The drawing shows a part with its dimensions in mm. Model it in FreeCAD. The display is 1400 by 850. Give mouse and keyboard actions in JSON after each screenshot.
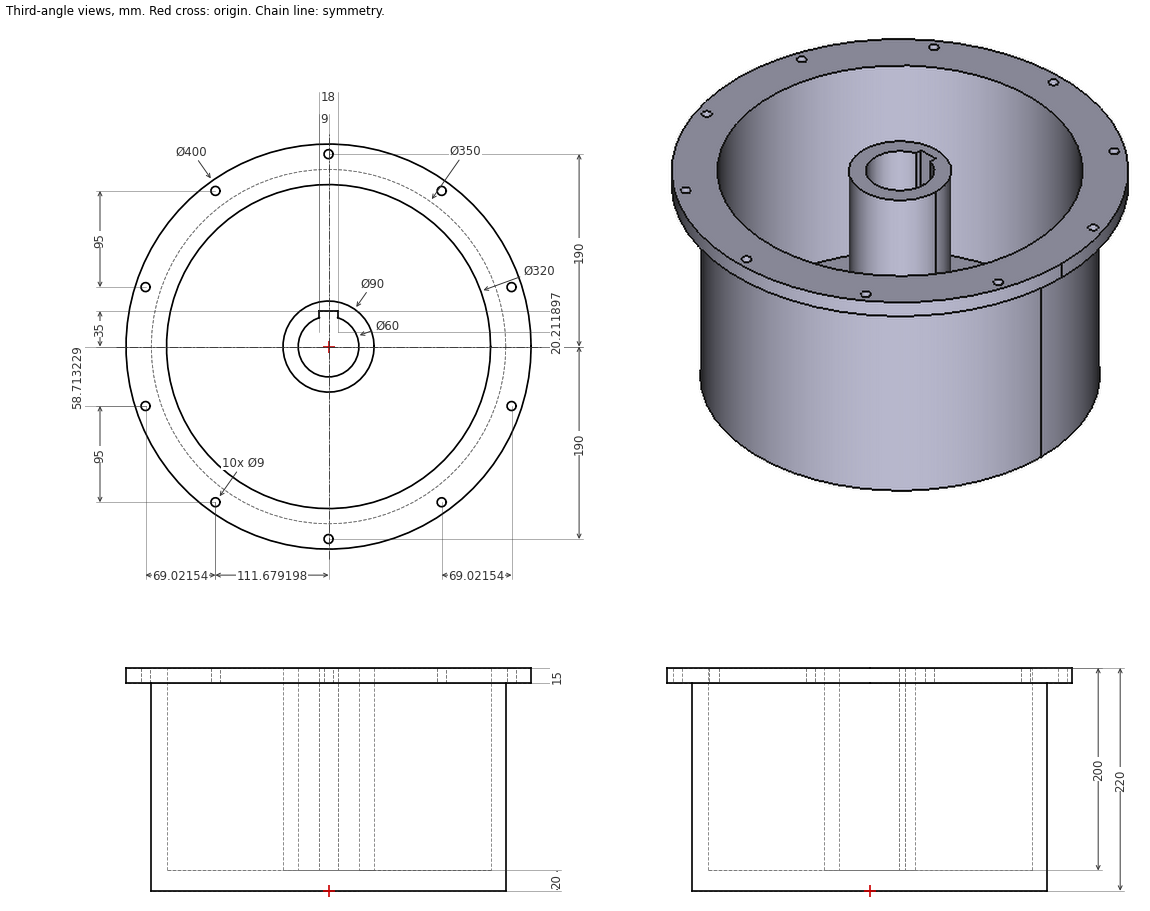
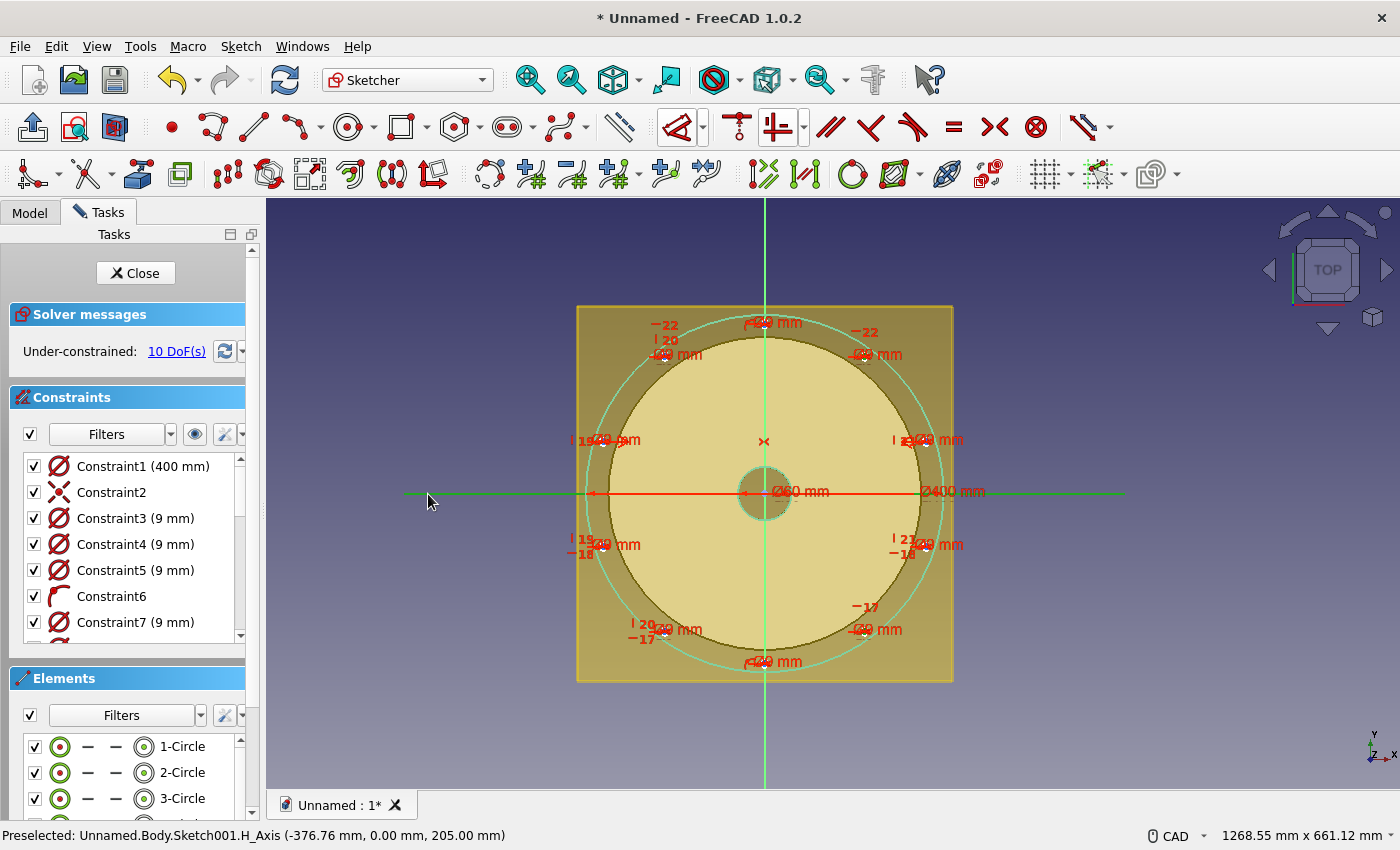
{"action": "left_click", "coordinate": [995, 128]}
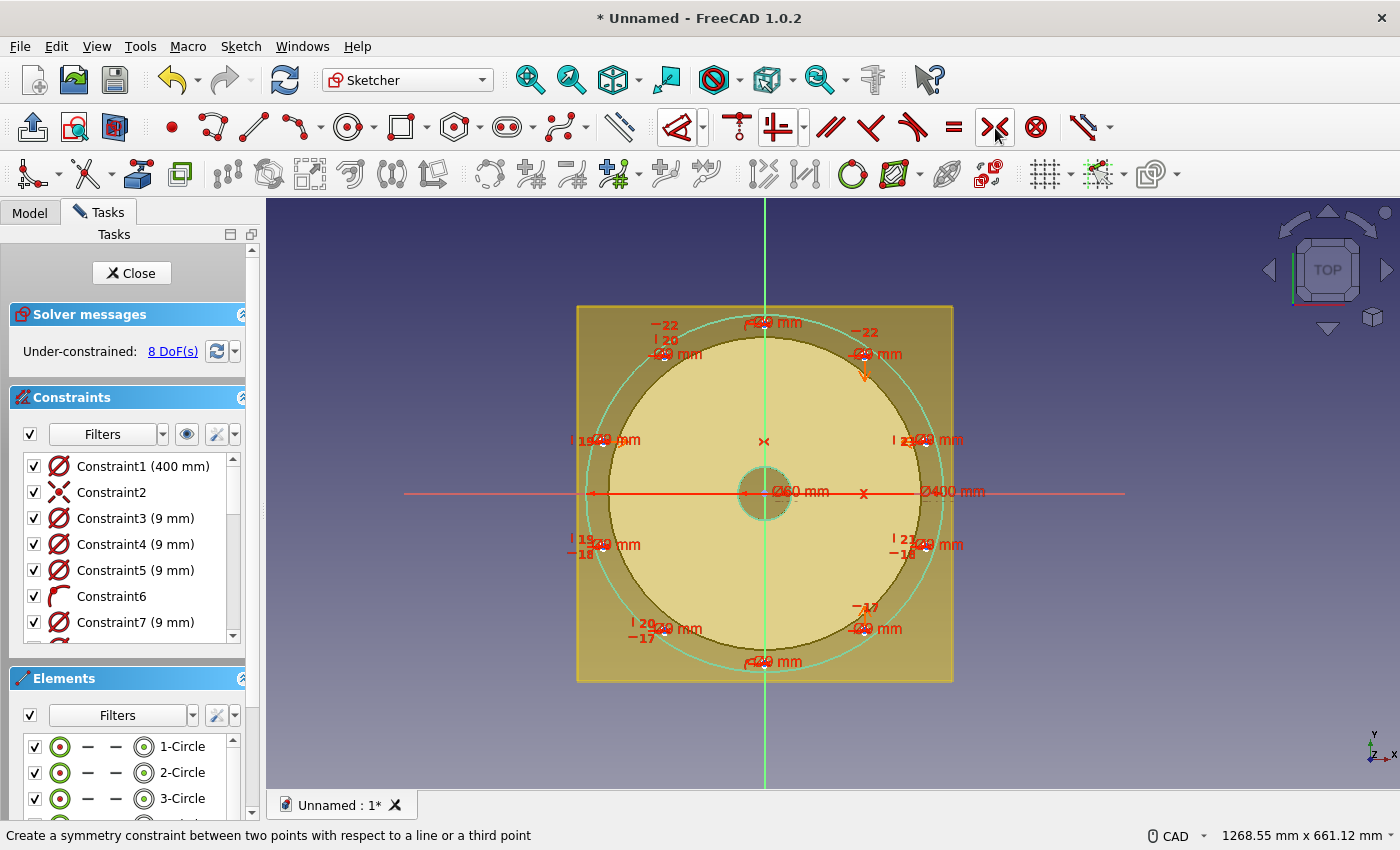
{"action": "left_click", "coordinate": [676, 128]}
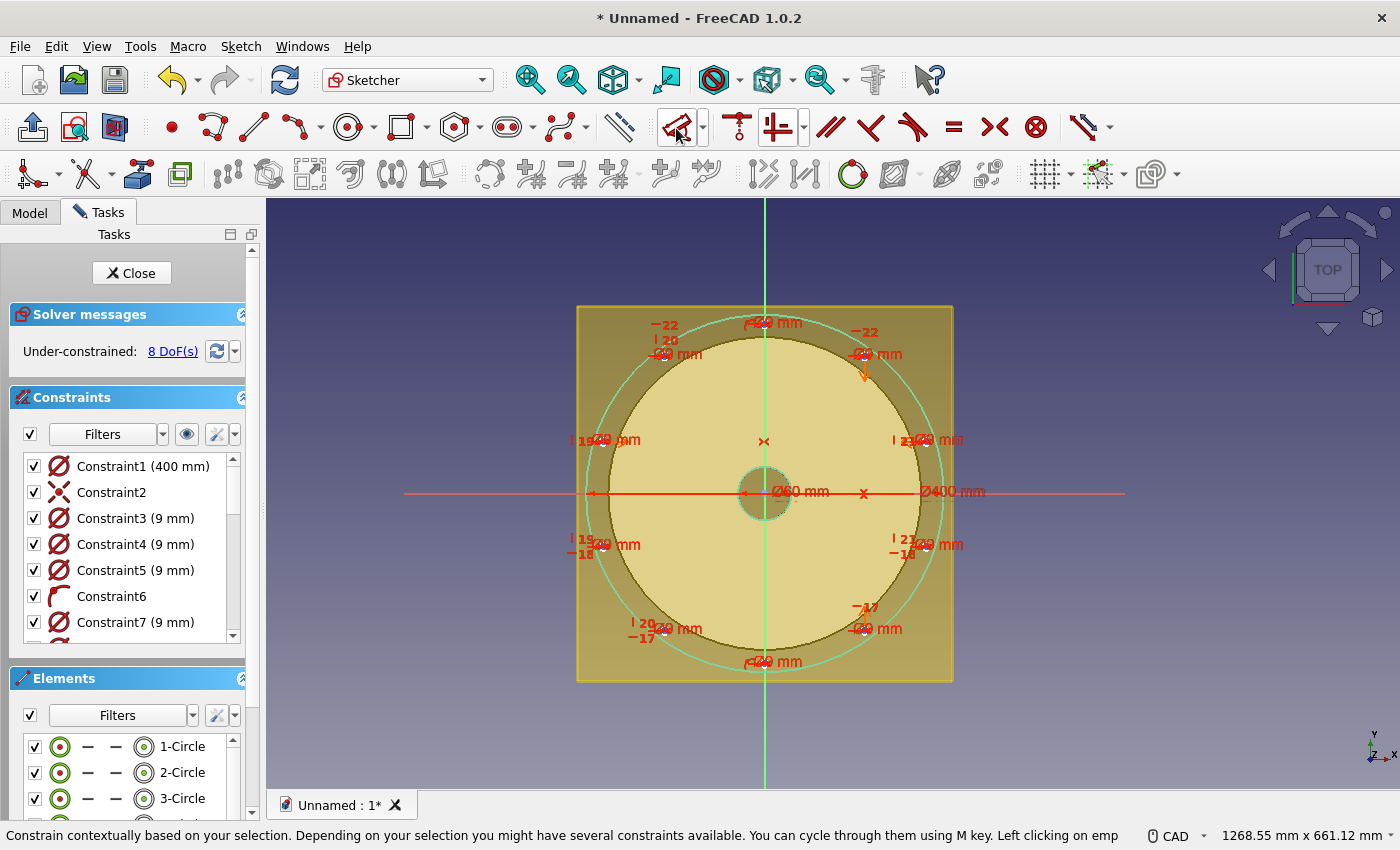
{"action": "left_click", "coordinate": [765, 664]}
{"action": "left_click", "coordinate": [799, 579]}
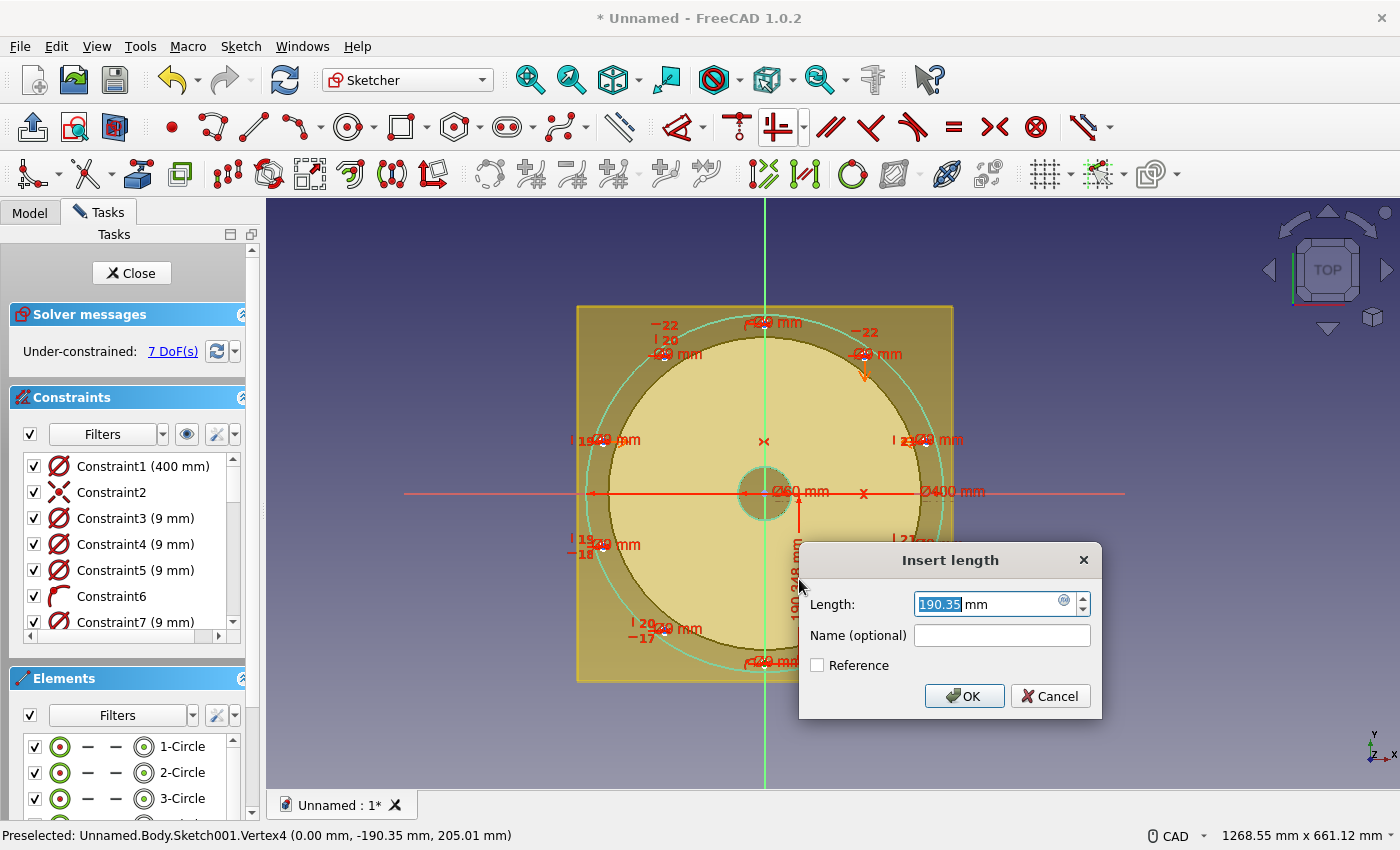
{"action": "type", "text": "190"}
{"action": "key", "text": "Return"}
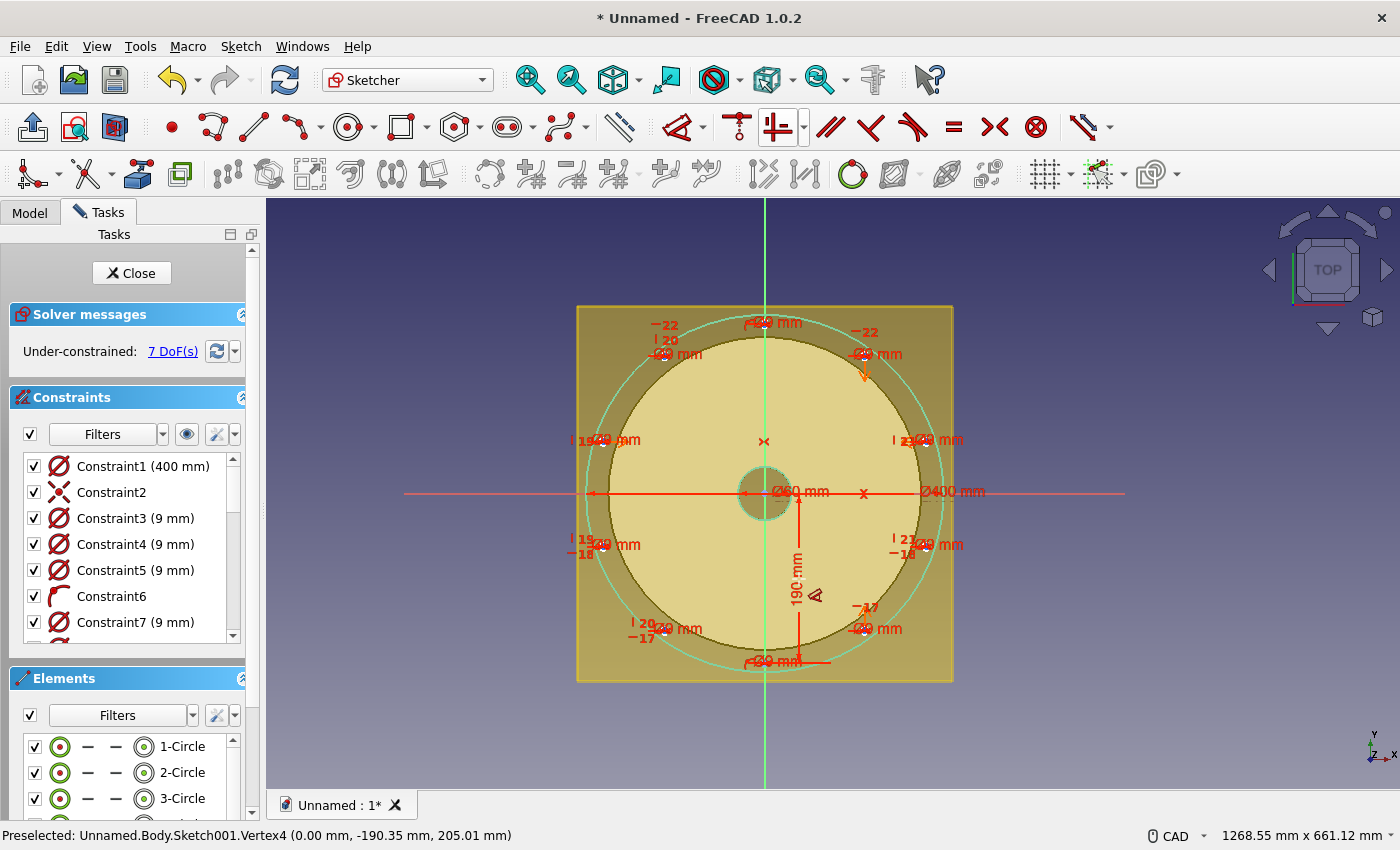
{"action": "left_click", "coordinate": [765, 324]}
{"action": "left_click", "coordinate": [799, 409]}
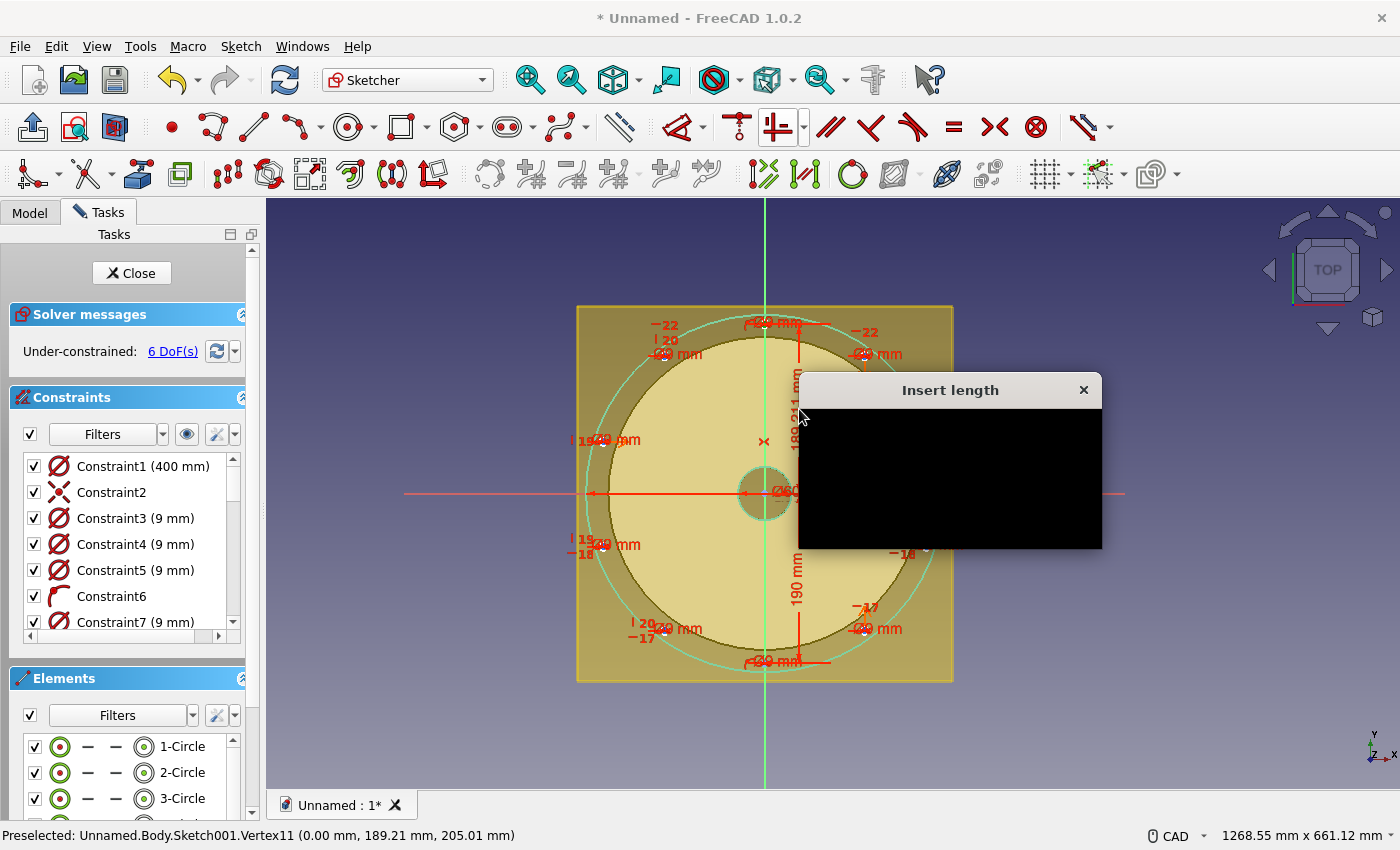
{"action": "type", "text": "190"}
{"action": "key", "text": "Return"}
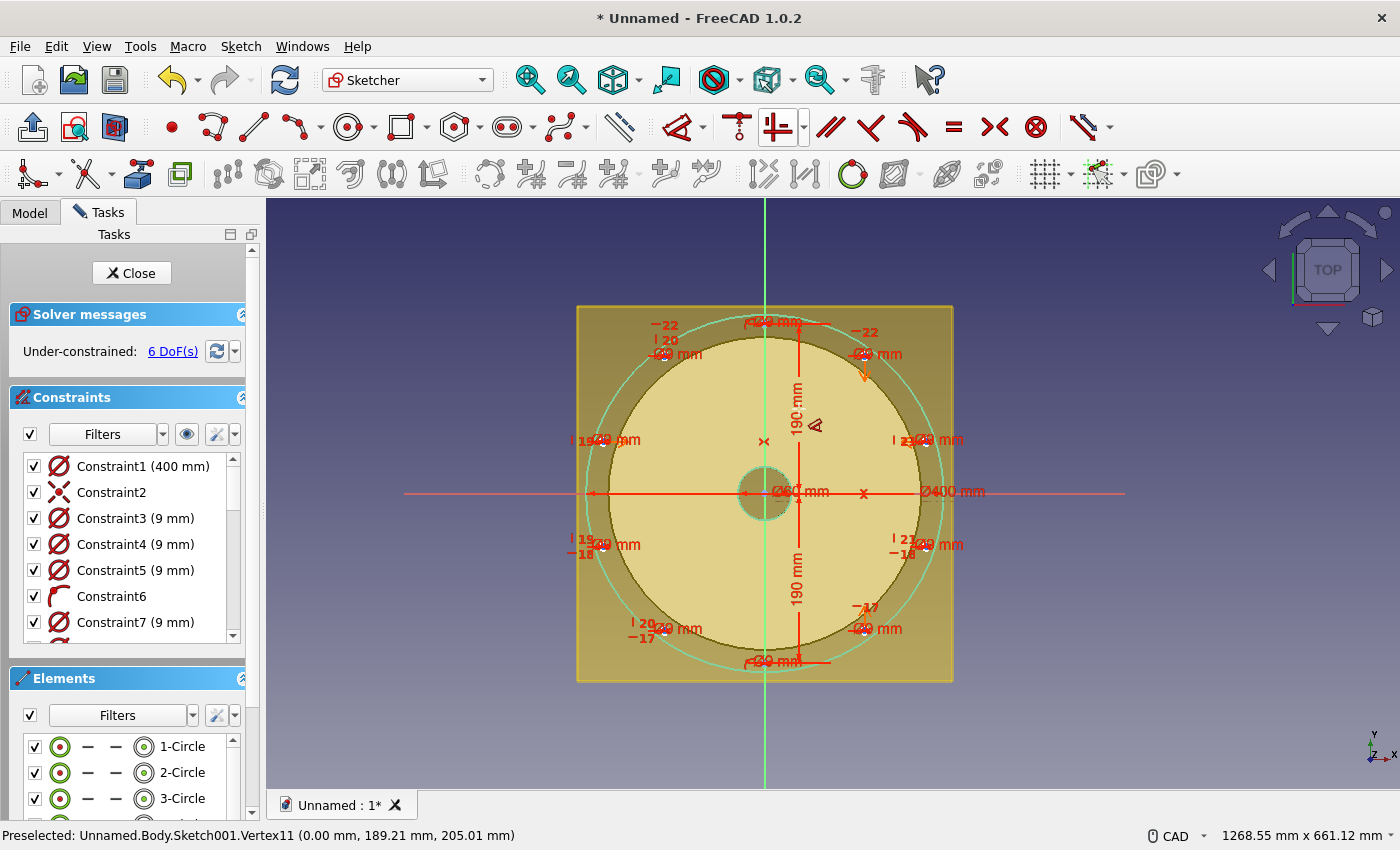
{"action": "left_click", "coordinate": [665, 631]}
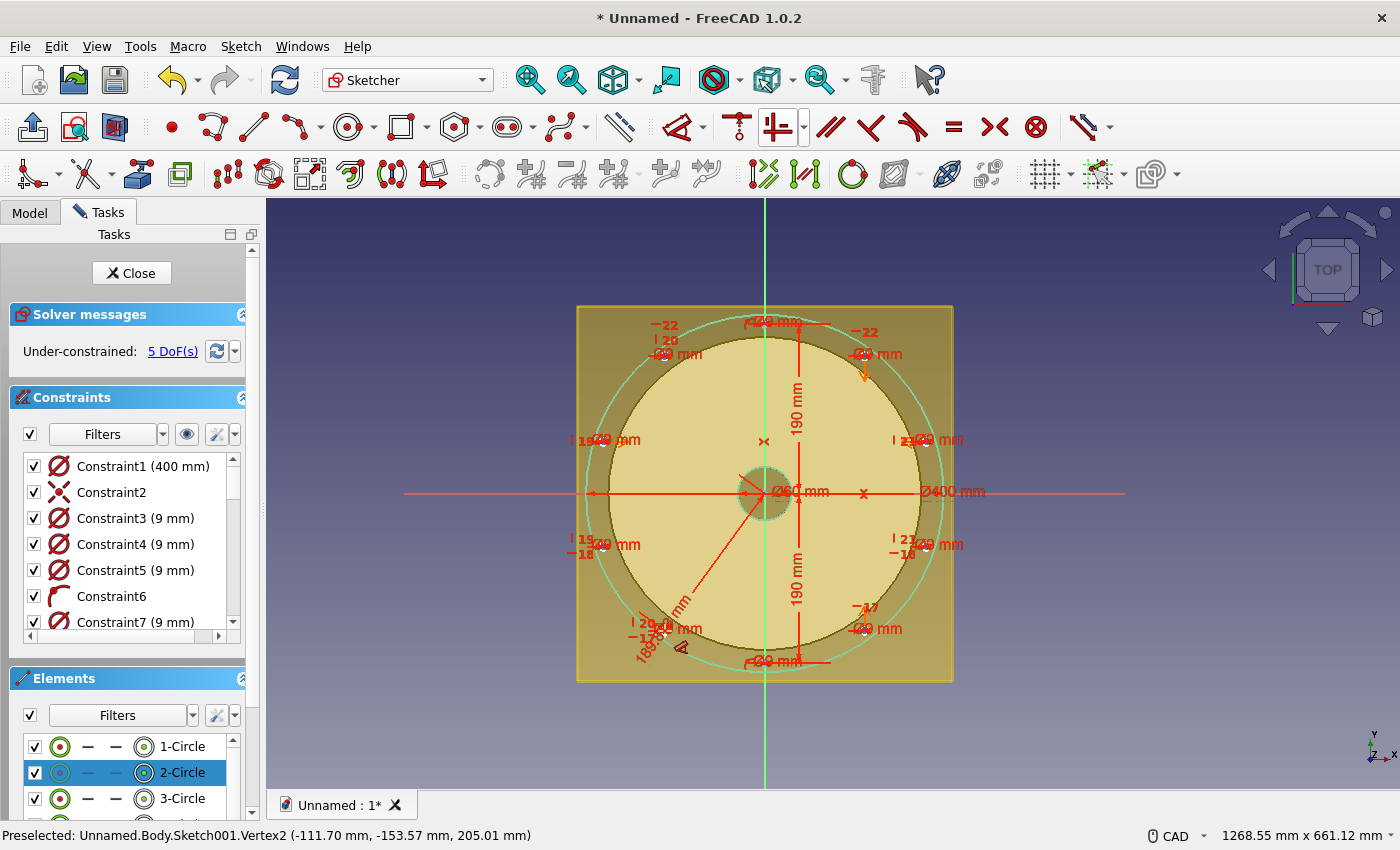
{"action": "left_click", "coordinate": [603, 547]}
{"action": "left_click", "coordinate": [569, 589]}